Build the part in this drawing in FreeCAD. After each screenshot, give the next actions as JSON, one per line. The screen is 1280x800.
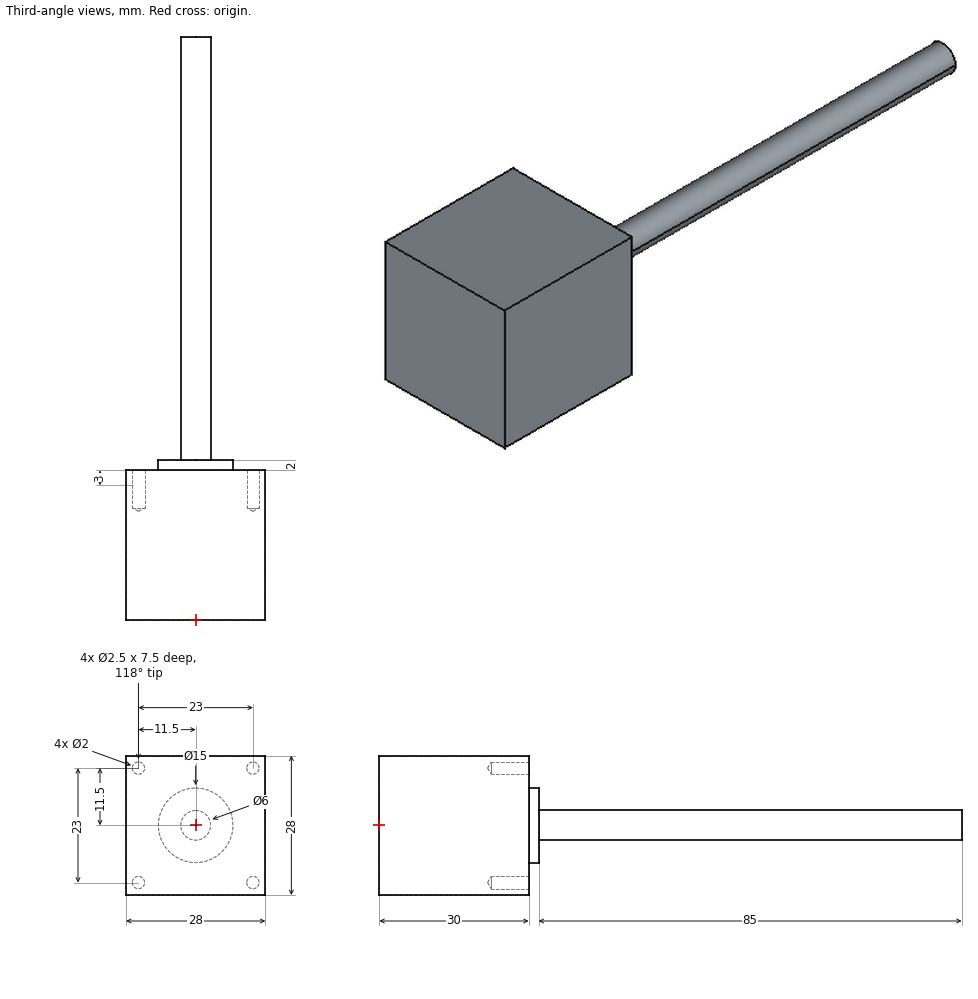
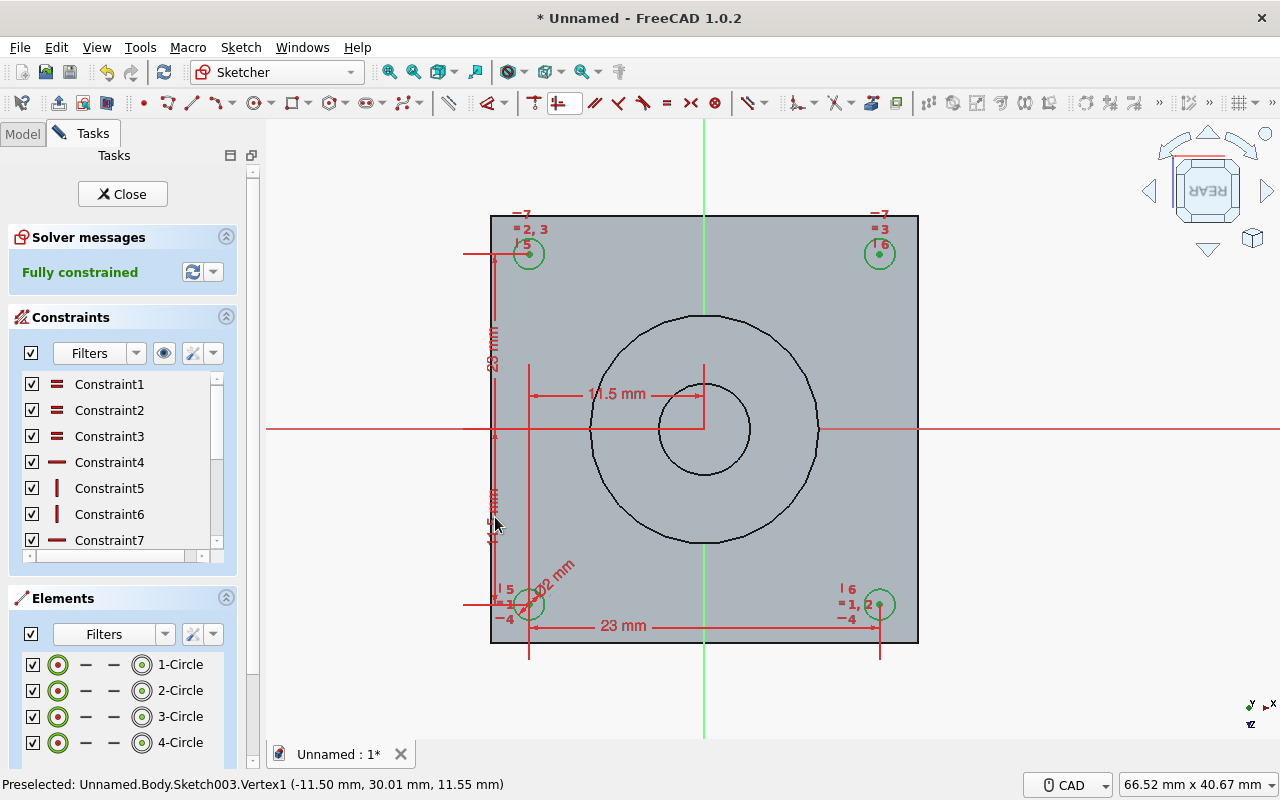
{"action": "left_click", "coordinate": [123, 194]}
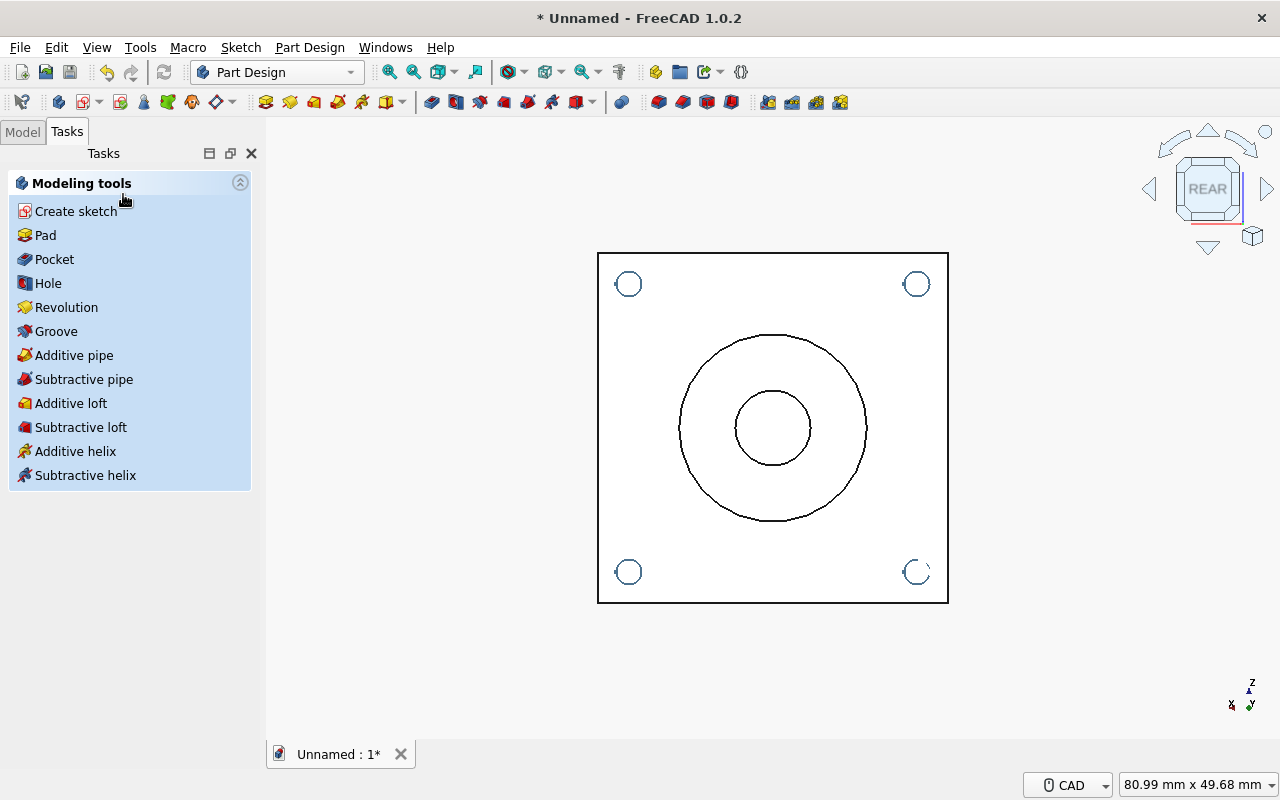
{"action": "left_click", "coordinate": [432, 102]}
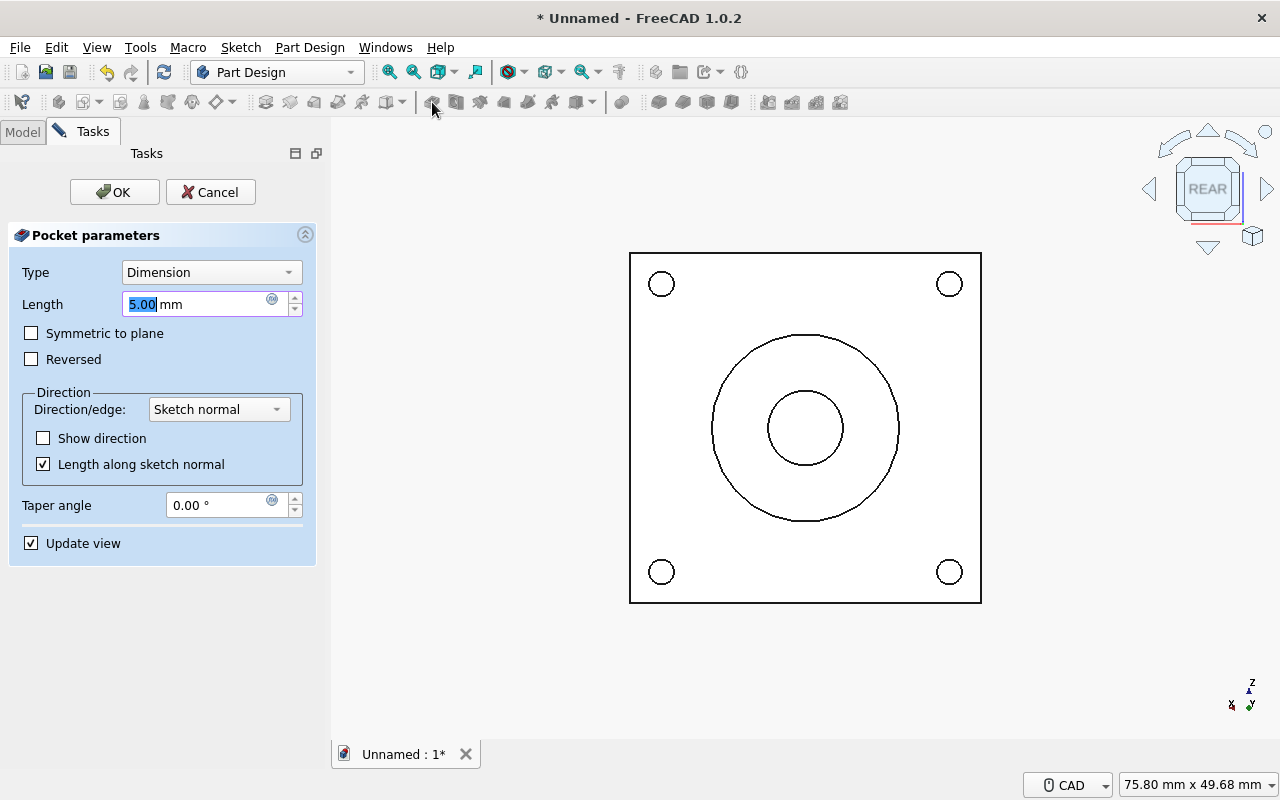
{"action": "type", "text": "3"}
{"action": "key", "text": "Tab"}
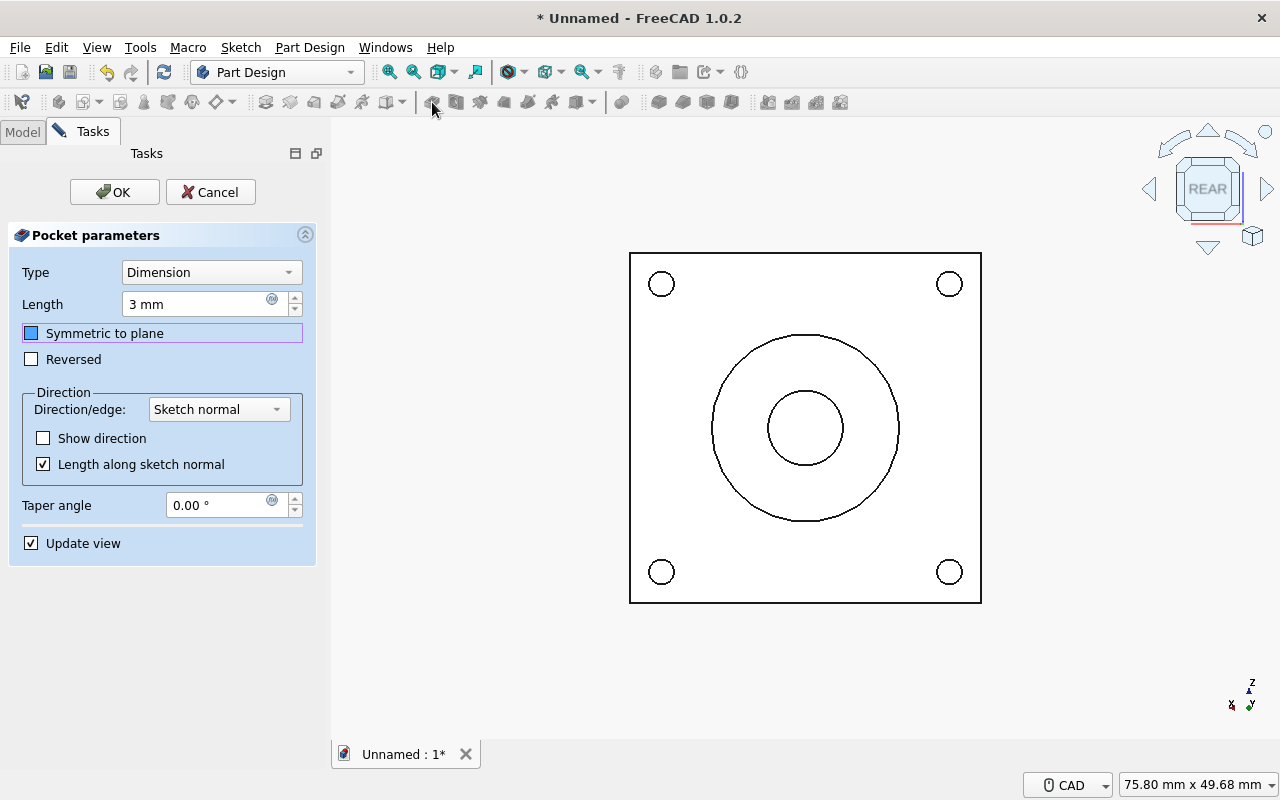
{"action": "left_click", "coordinate": [115, 192]}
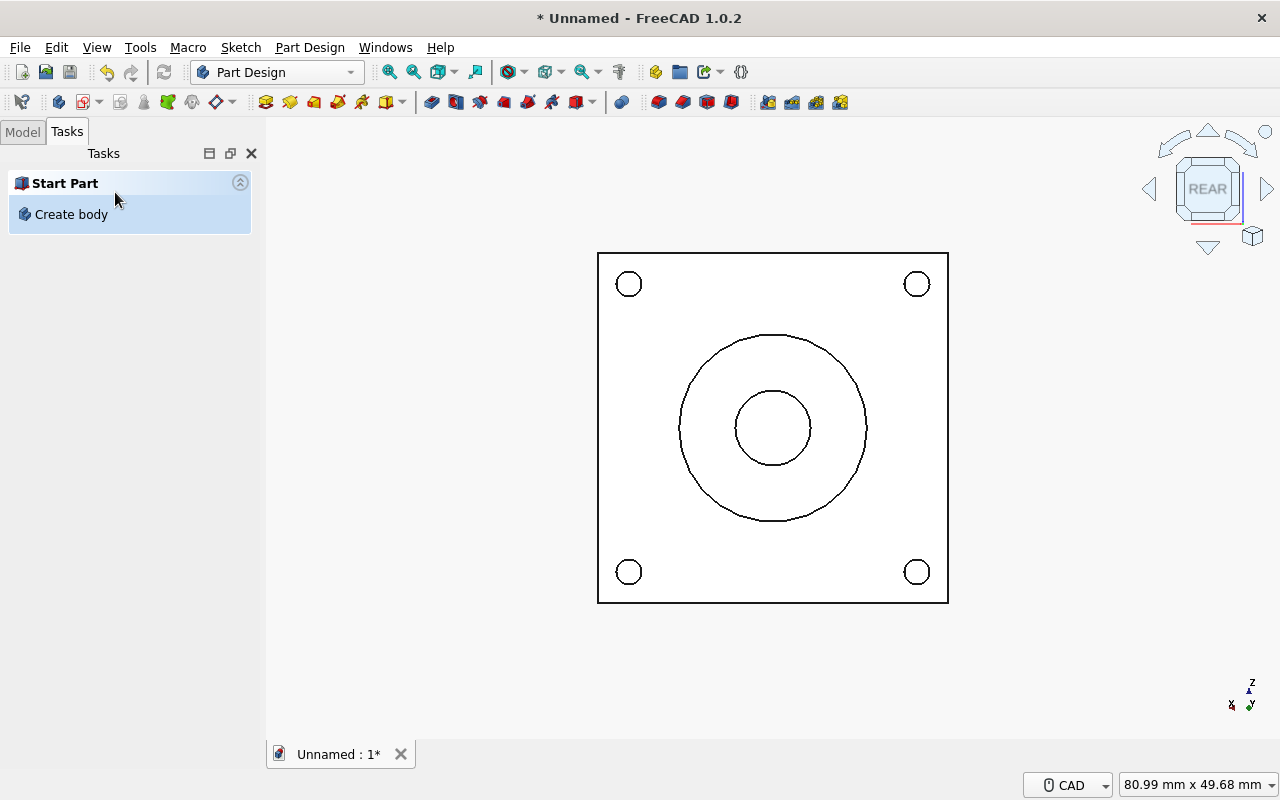
{"action": "left_click", "coordinate": [673, 527]}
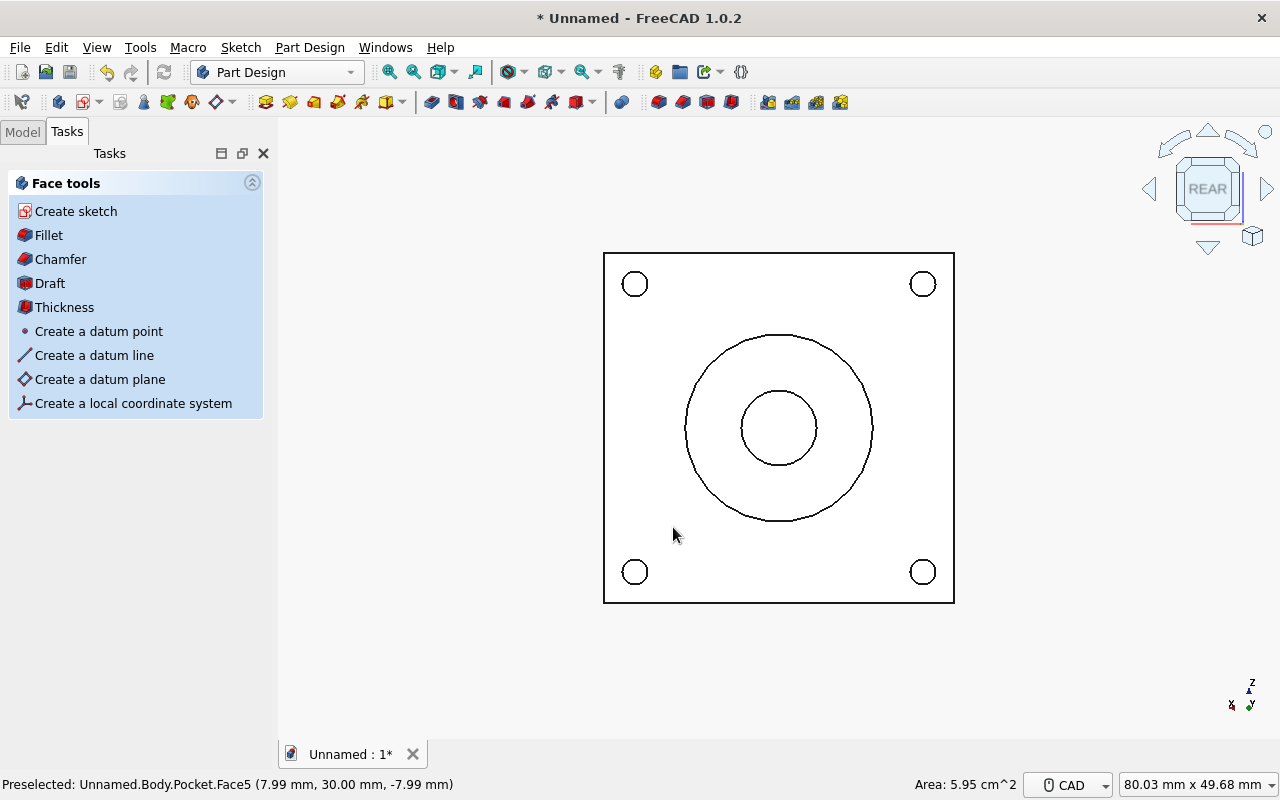
{"action": "left_click", "coordinate": [84, 102]}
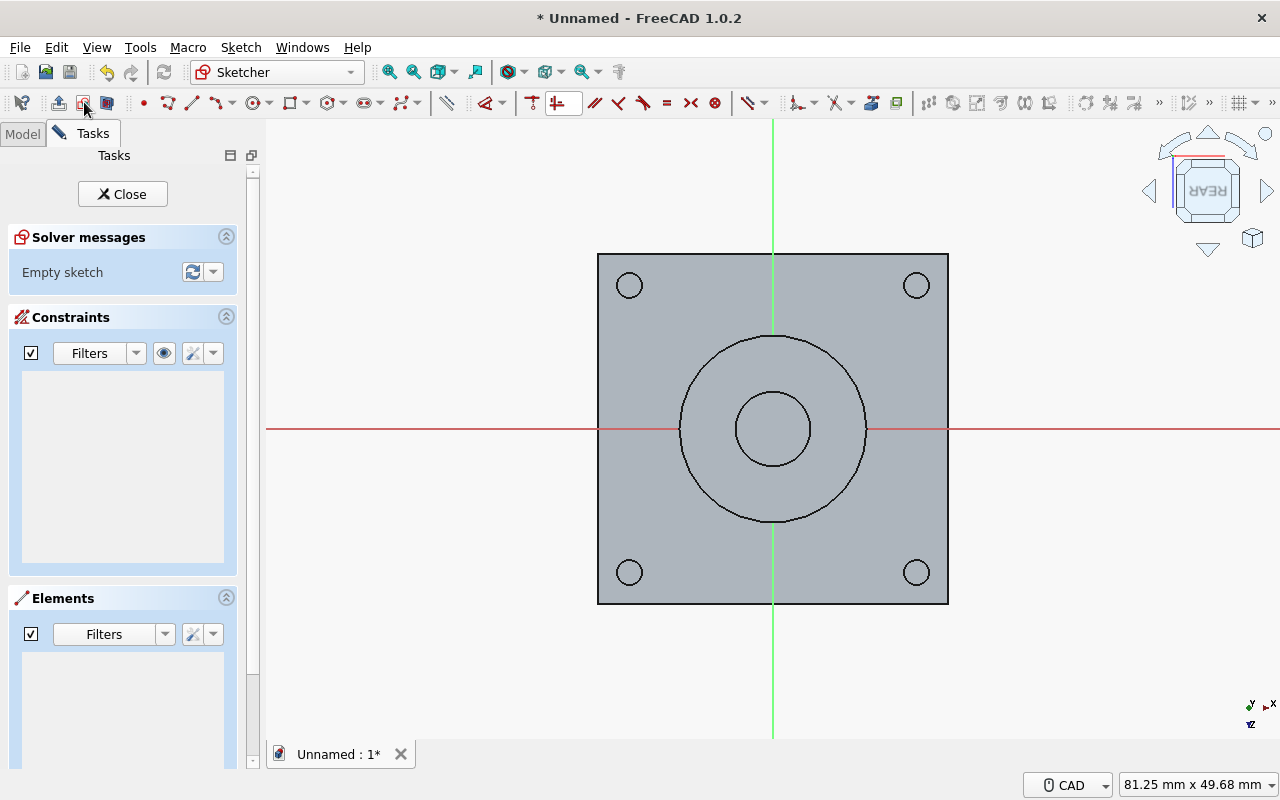
{"action": "left_click", "coordinate": [108, 104]}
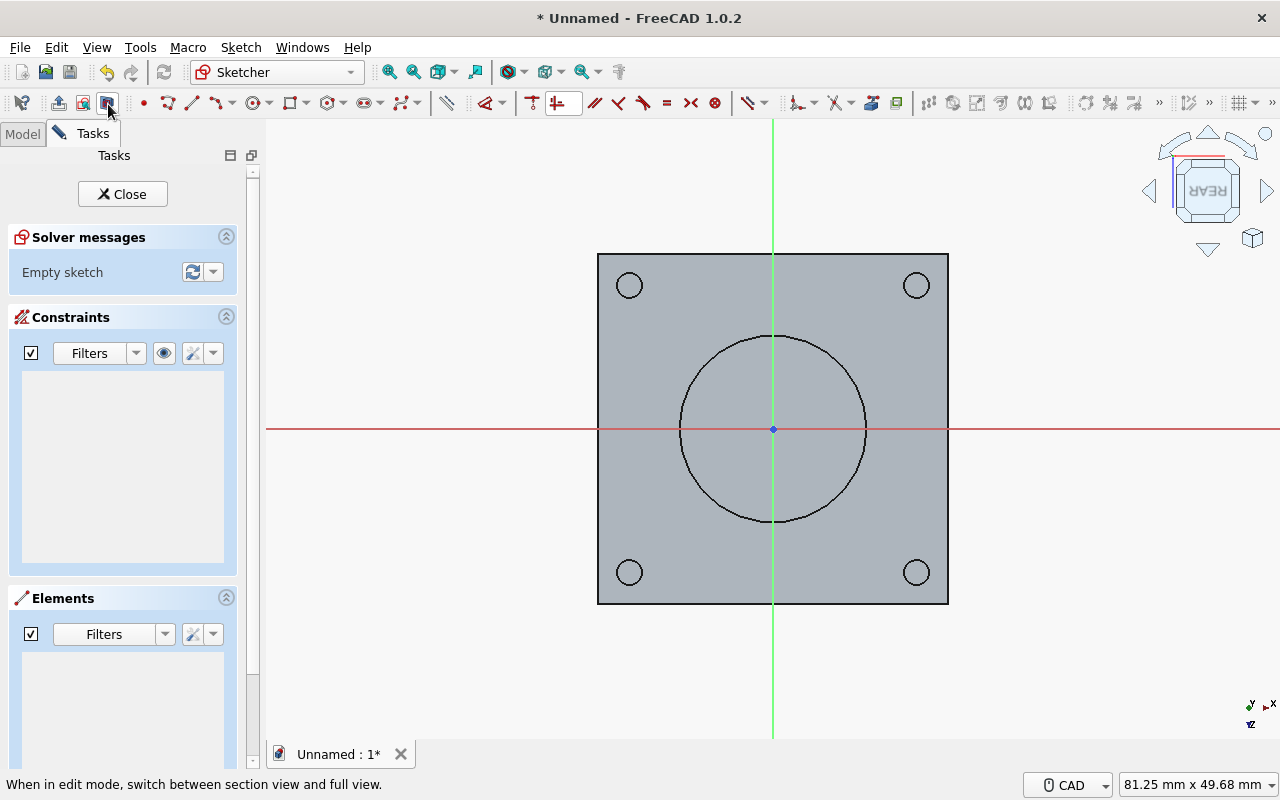
{"action": "left_click", "coordinate": [254, 104]}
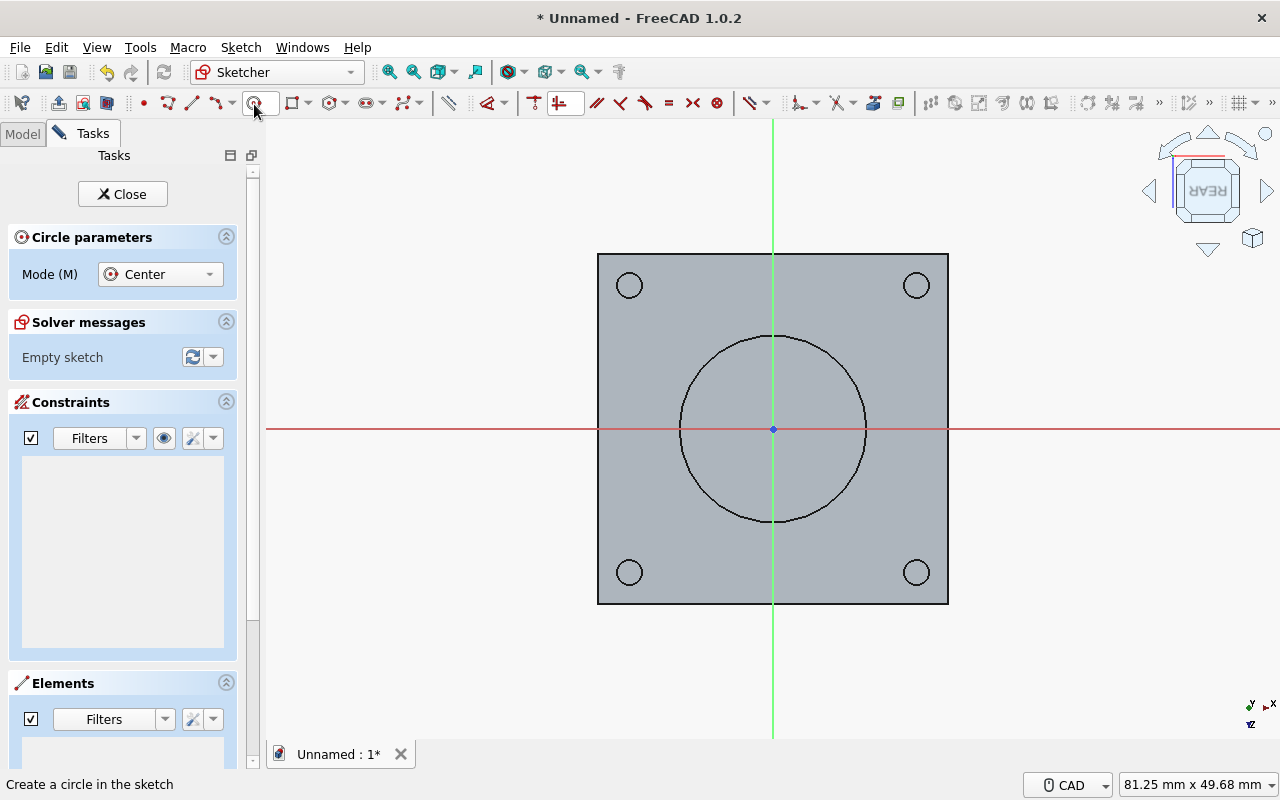
{"action": "scroll", "coordinate": [629, 573], "scroll_direction": "up", "scroll_amount": 2}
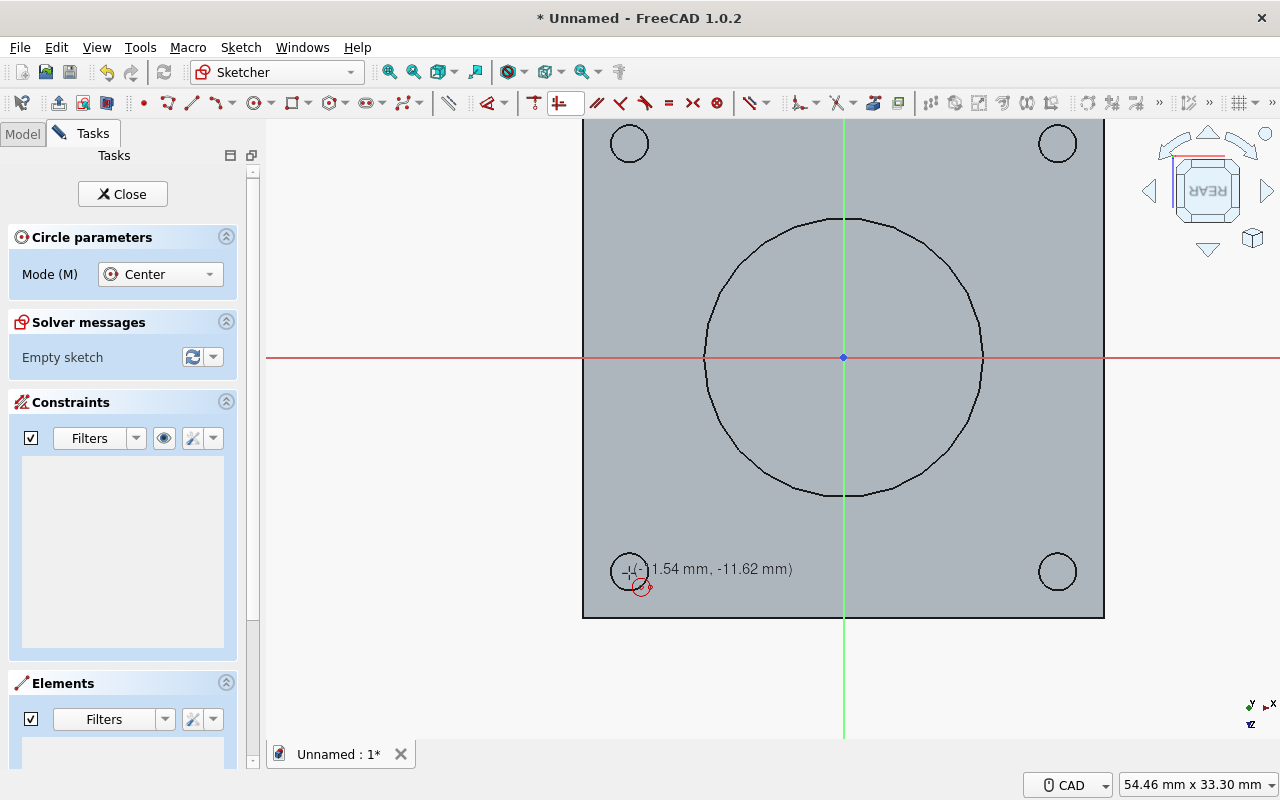
{"action": "left_click", "coordinate": [630, 572]}
{"action": "left_click", "coordinate": [646, 555]}